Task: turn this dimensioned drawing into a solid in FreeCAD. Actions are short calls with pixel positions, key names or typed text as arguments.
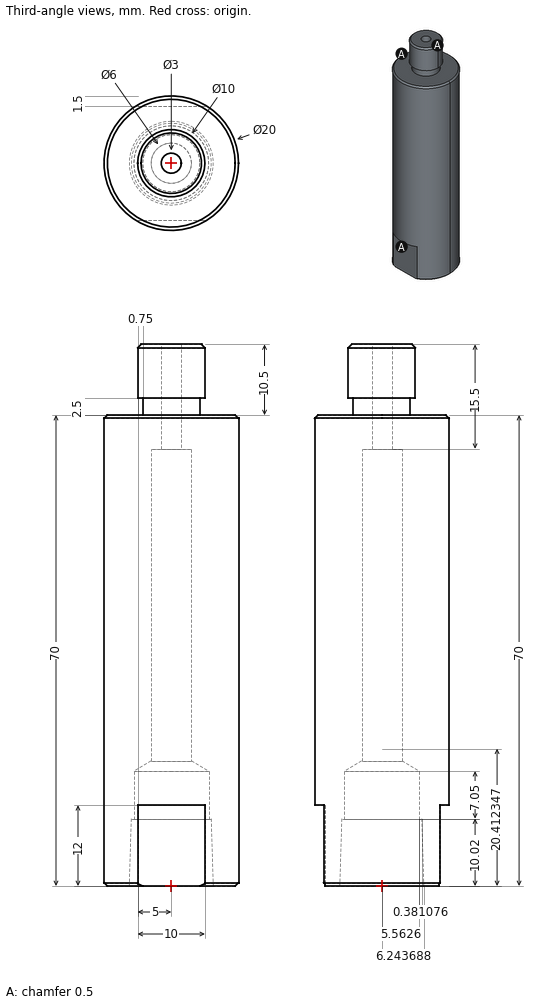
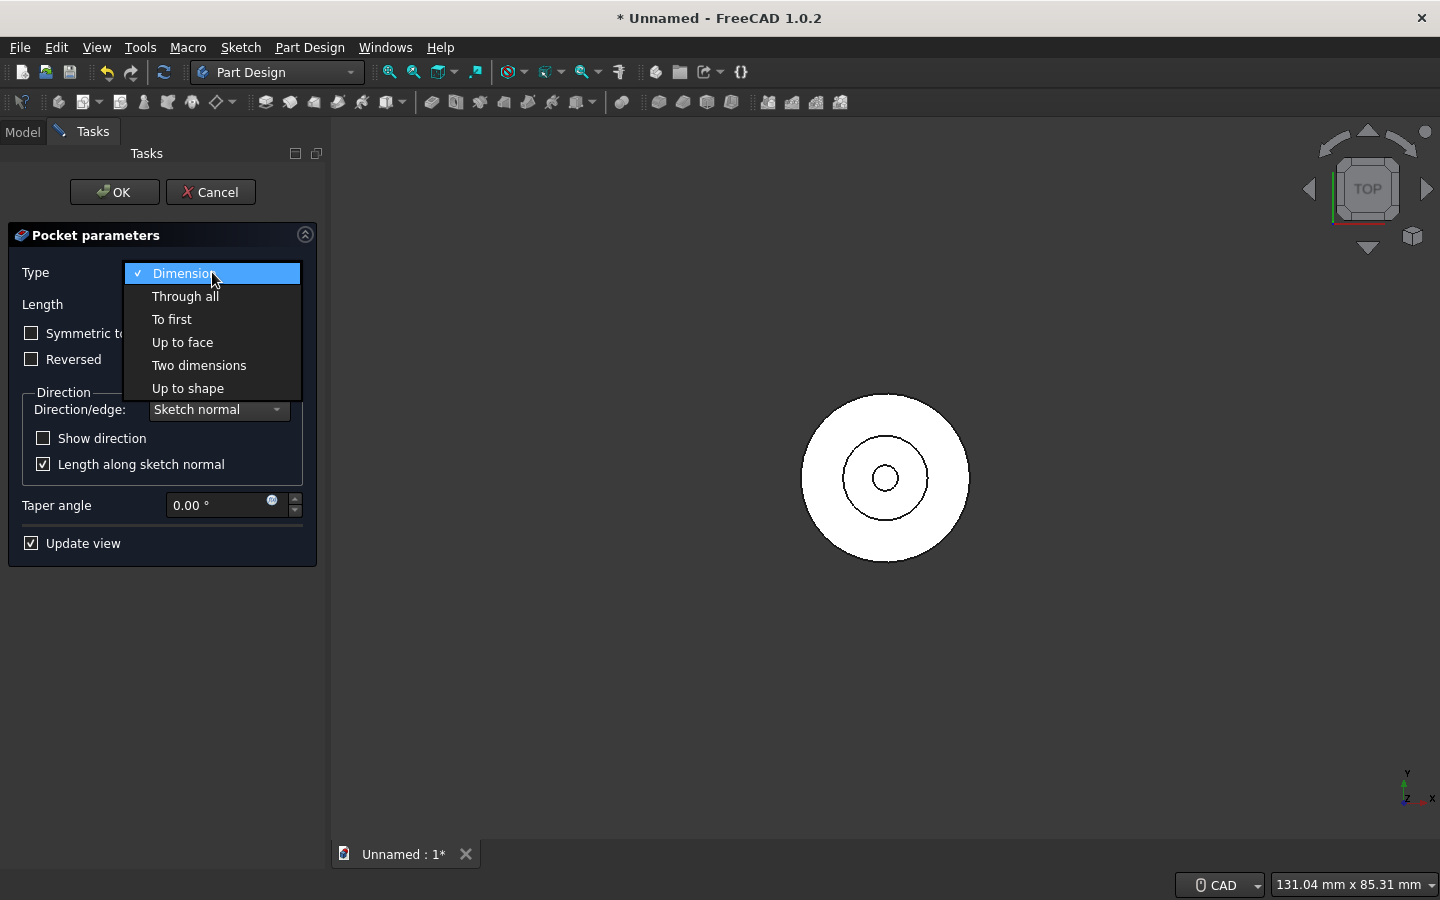
click(212, 320)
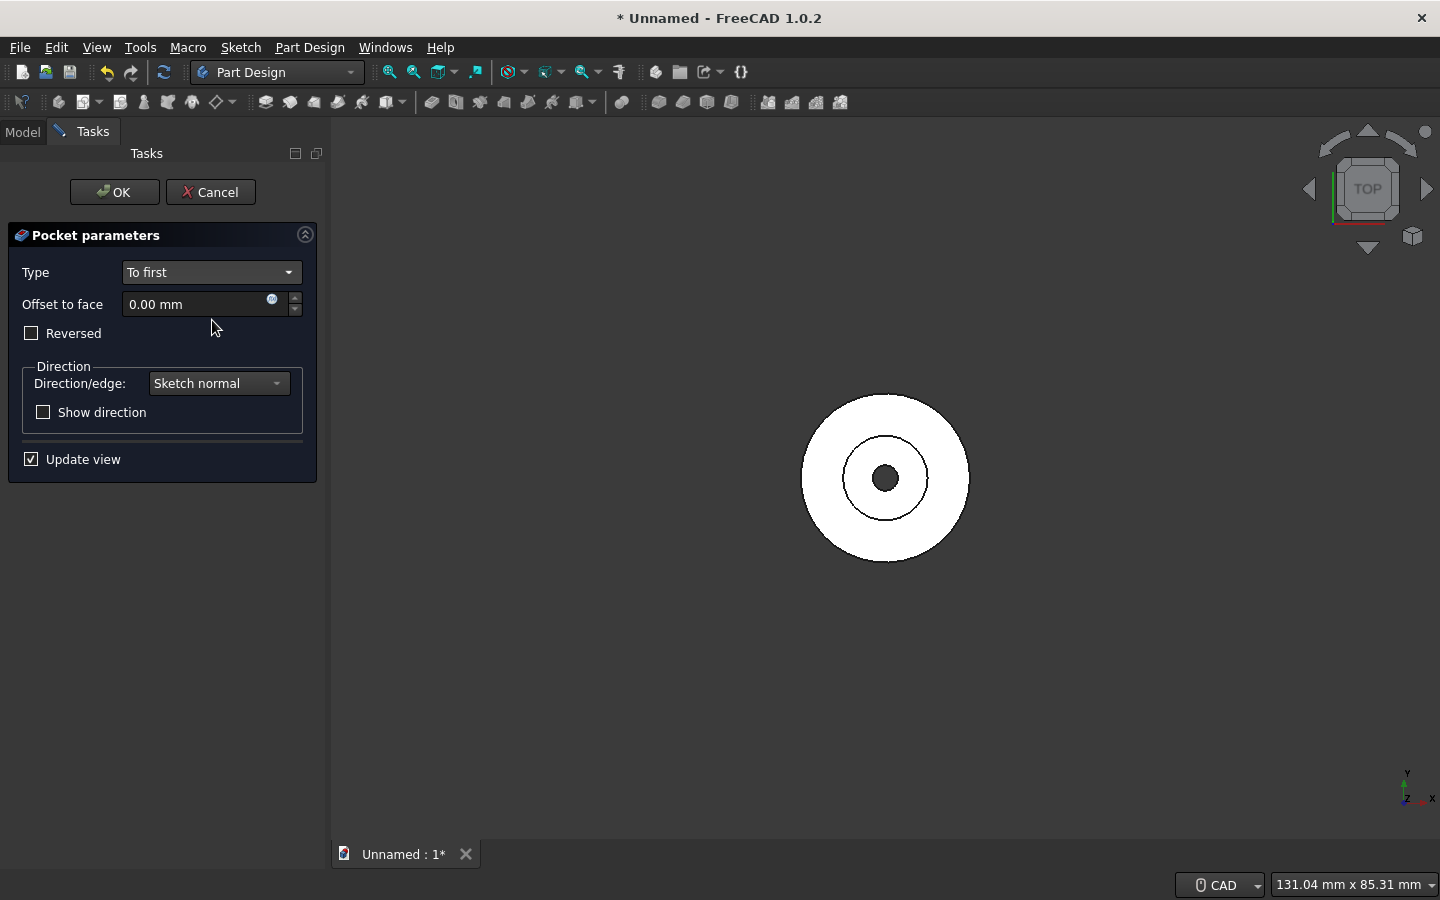
click(115, 192)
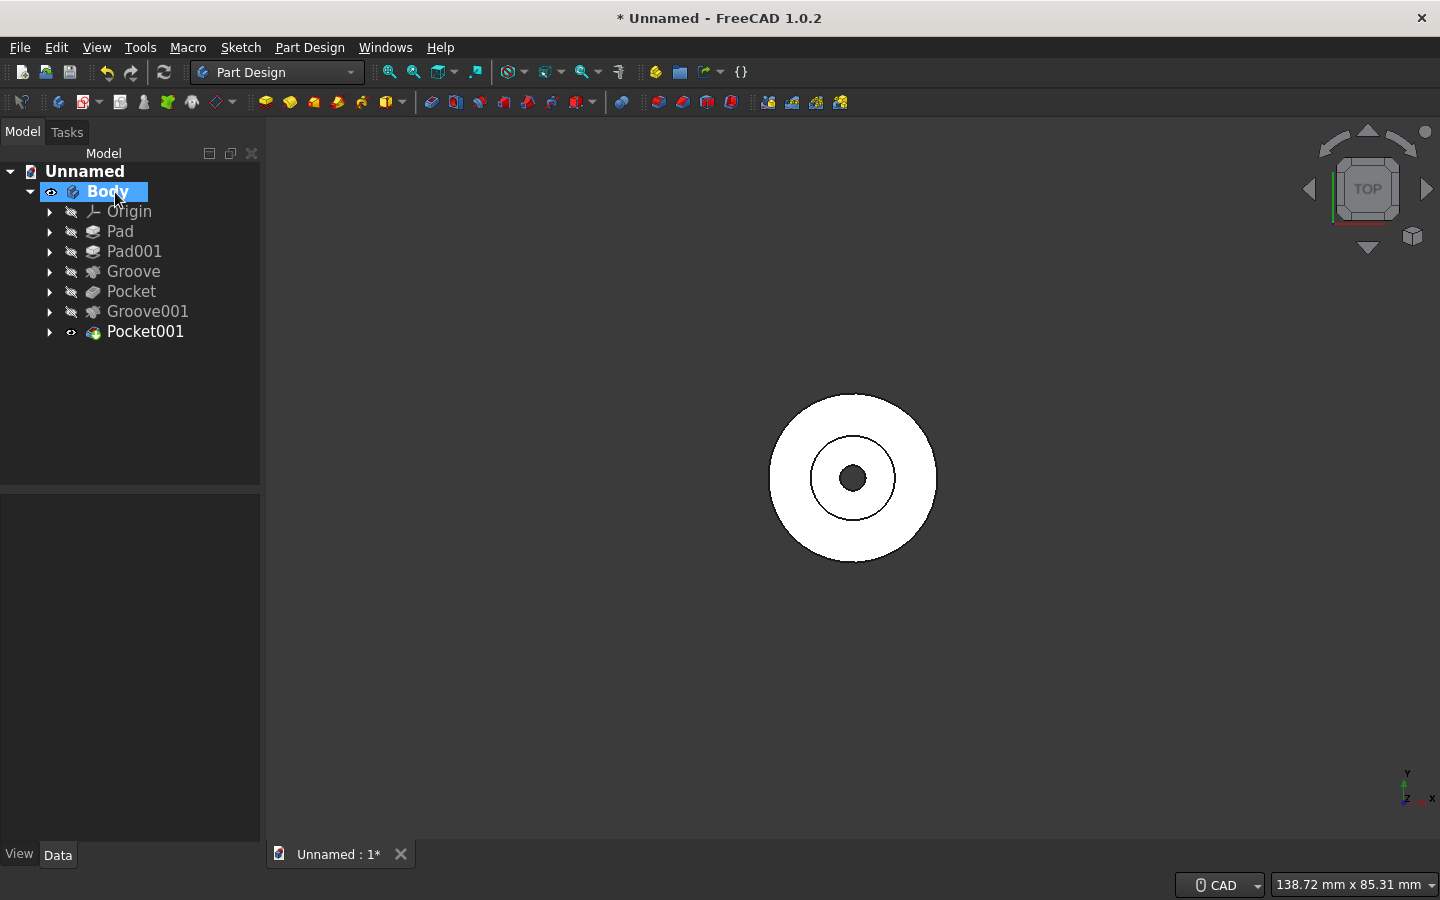
click(390, 72)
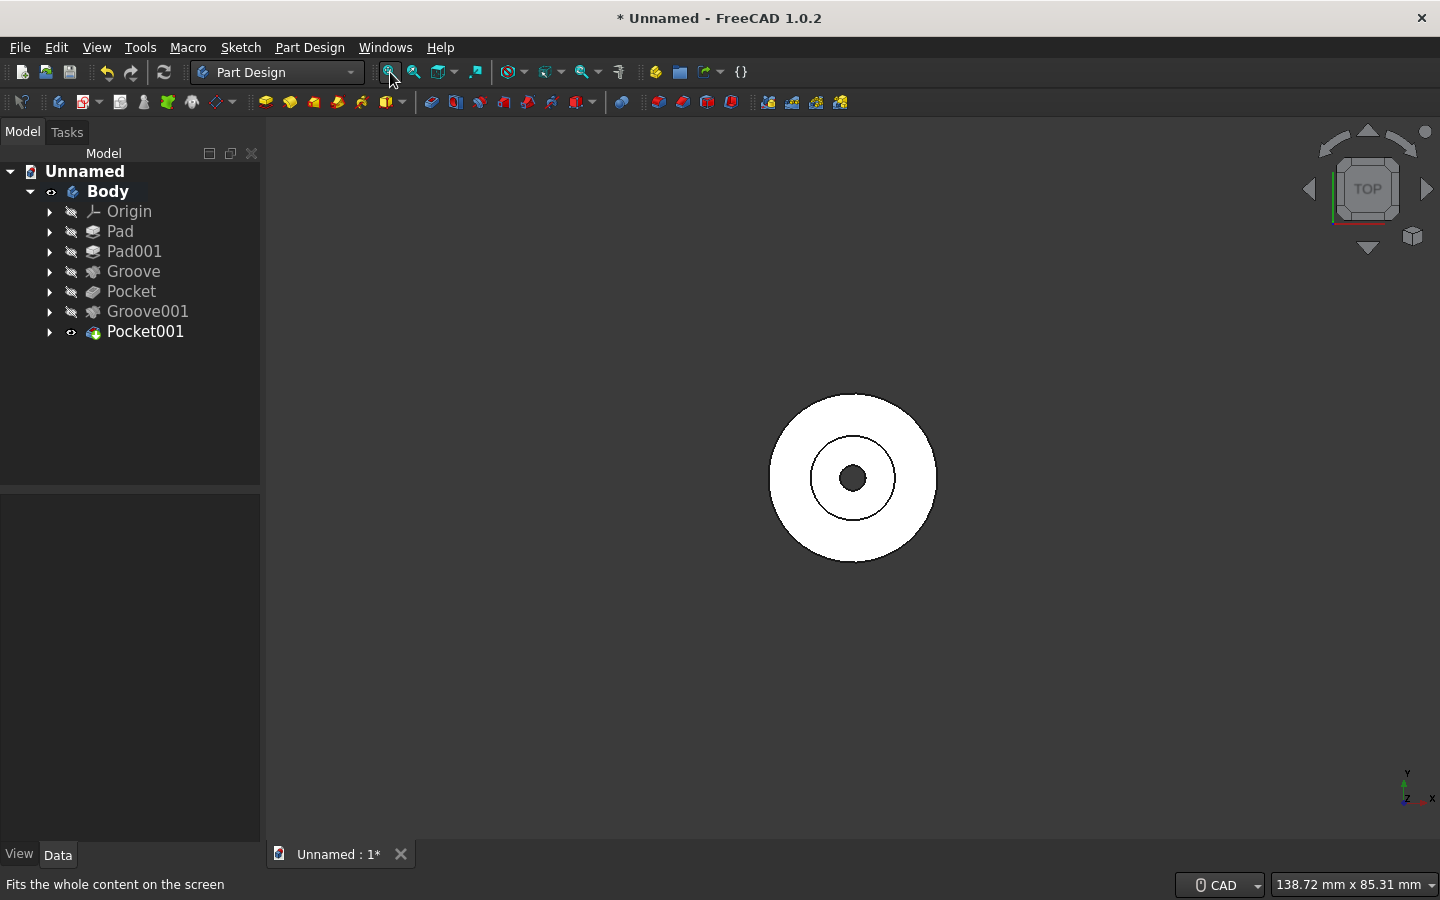
click(768, 477)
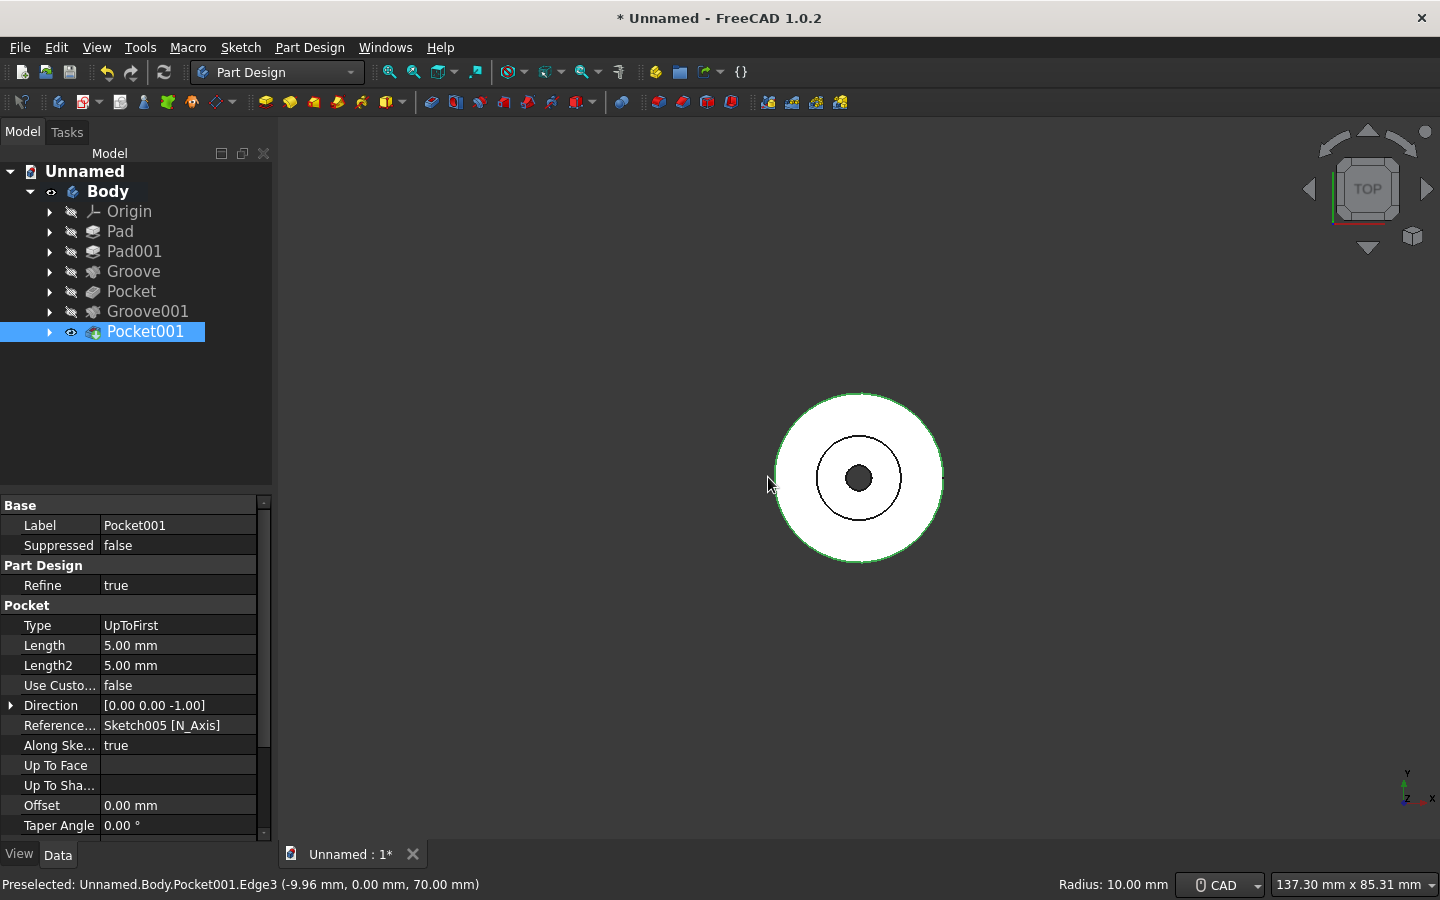
click(817, 477, ctrl)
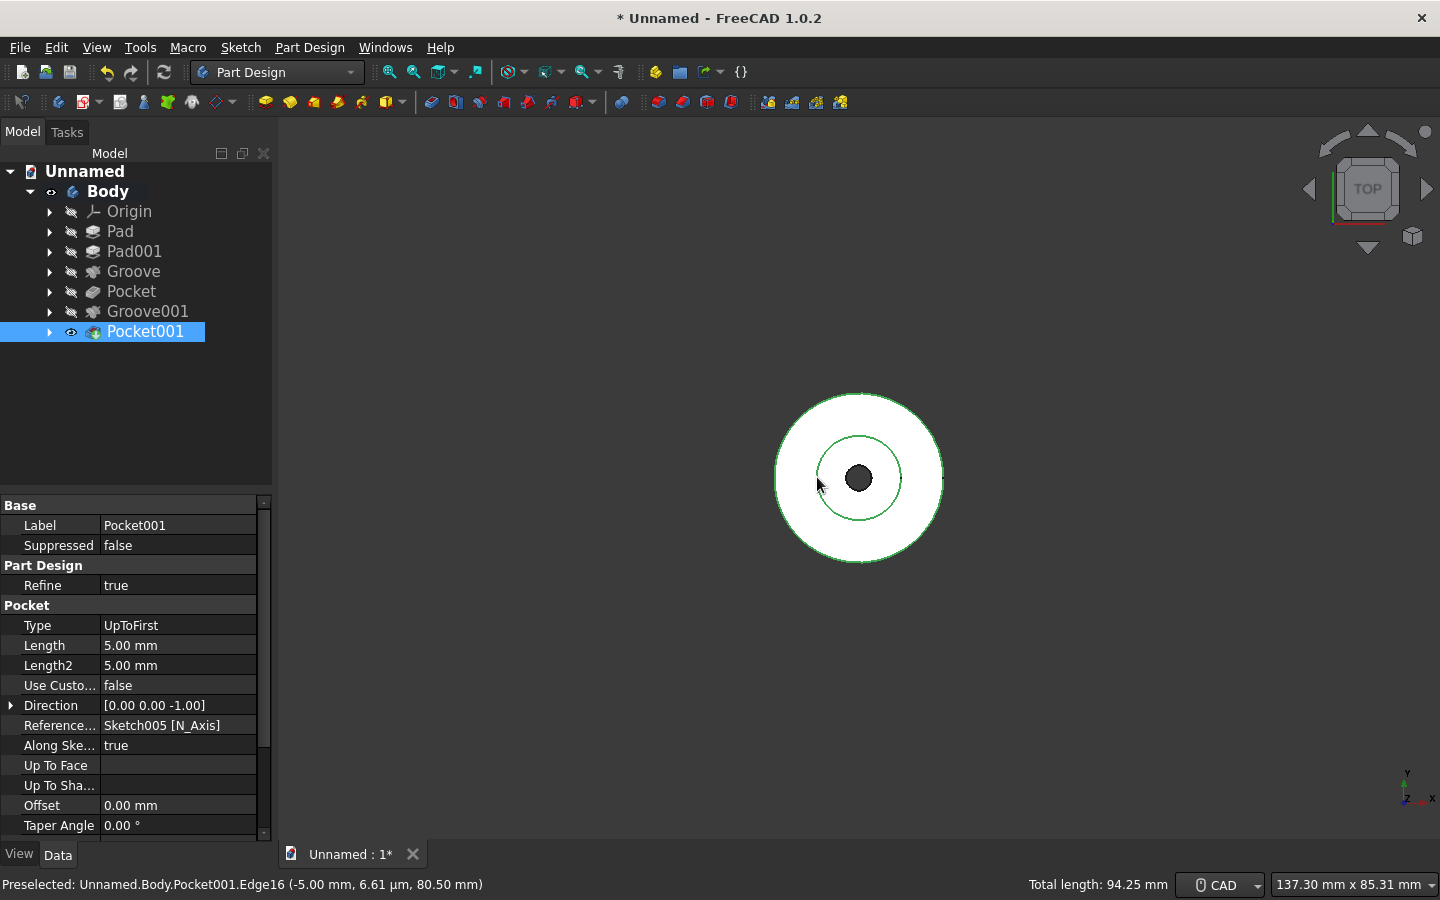
key(0)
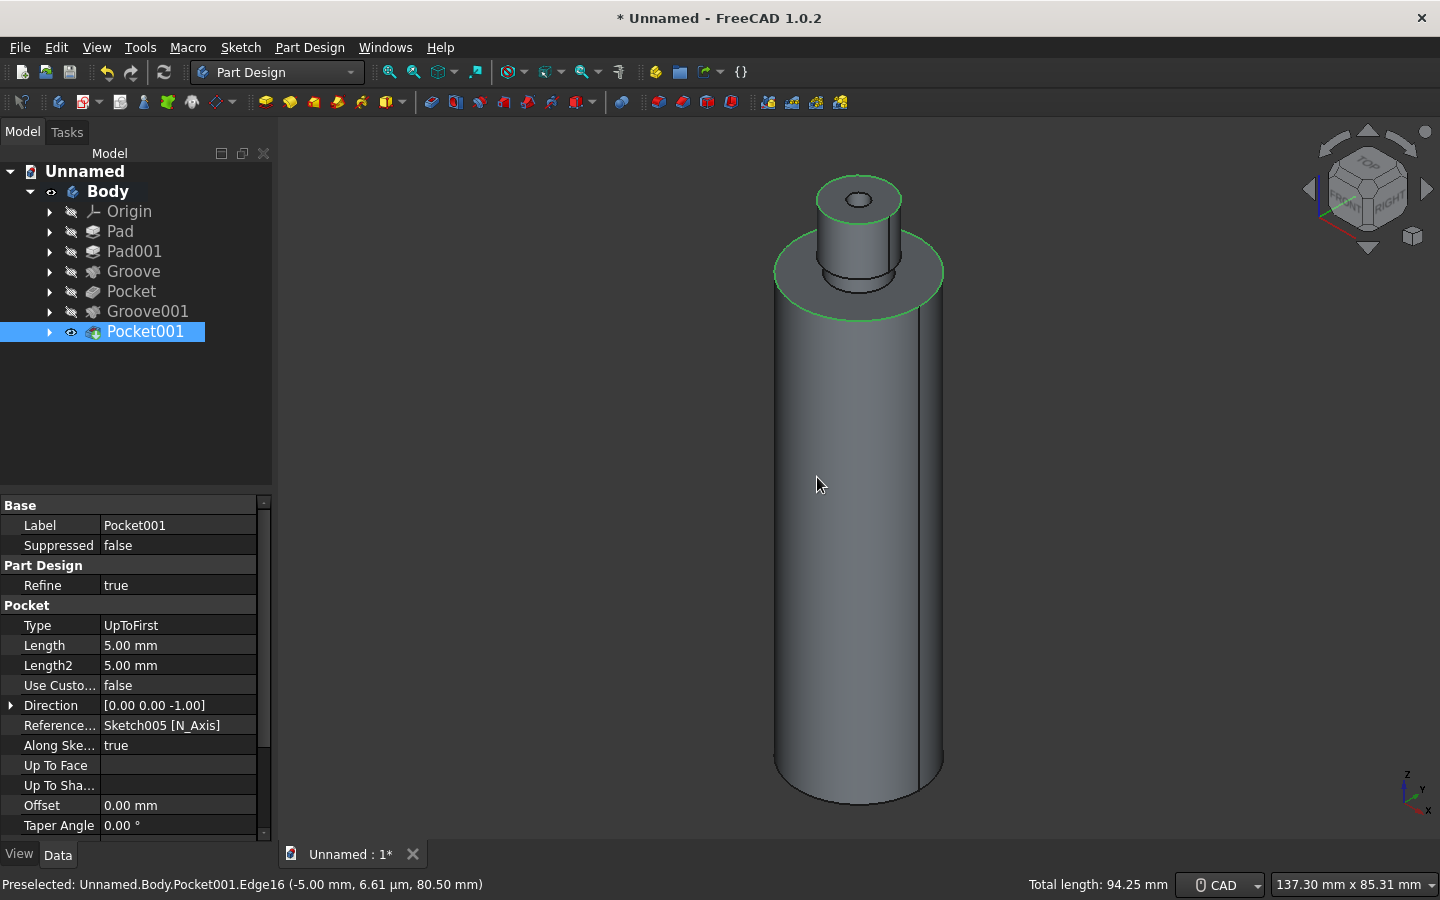
key(2)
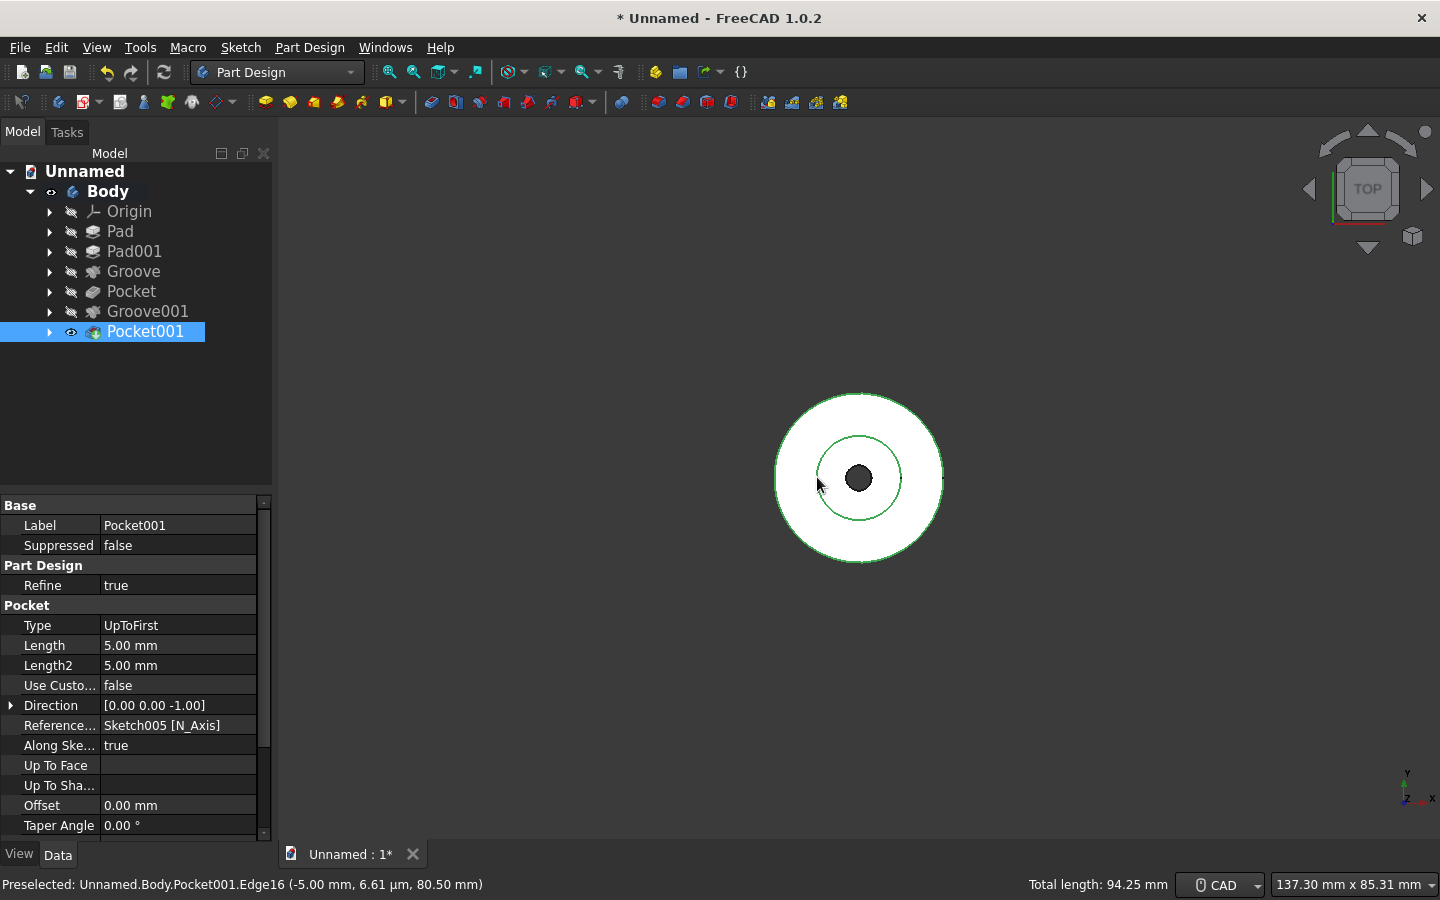
click(390, 72)